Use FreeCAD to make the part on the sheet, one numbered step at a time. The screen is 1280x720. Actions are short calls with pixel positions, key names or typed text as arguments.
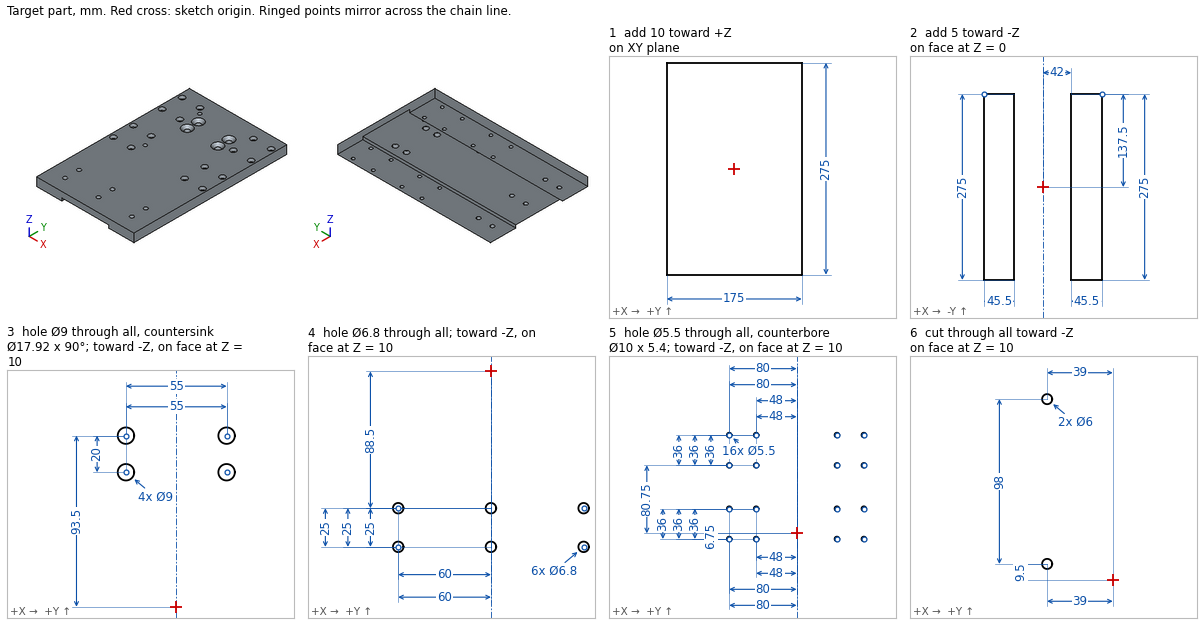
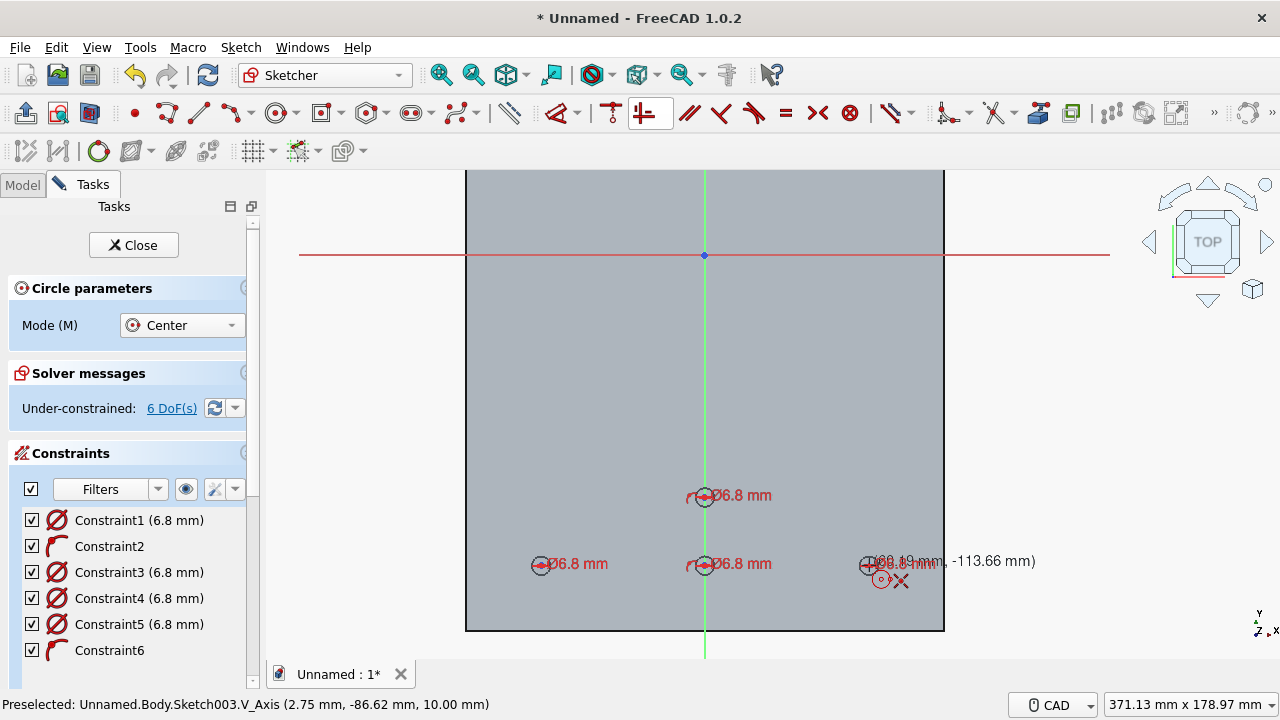
scroll(541, 497, up, 5)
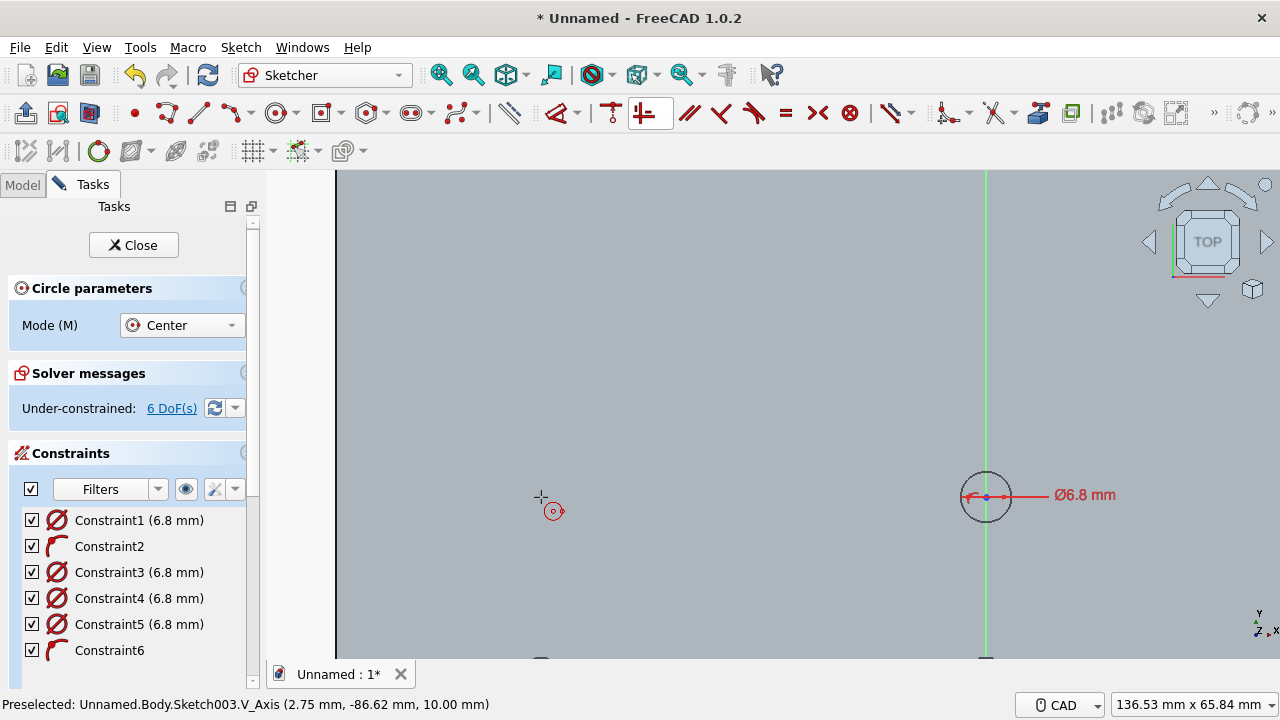
click(541, 496)
move(558, 478)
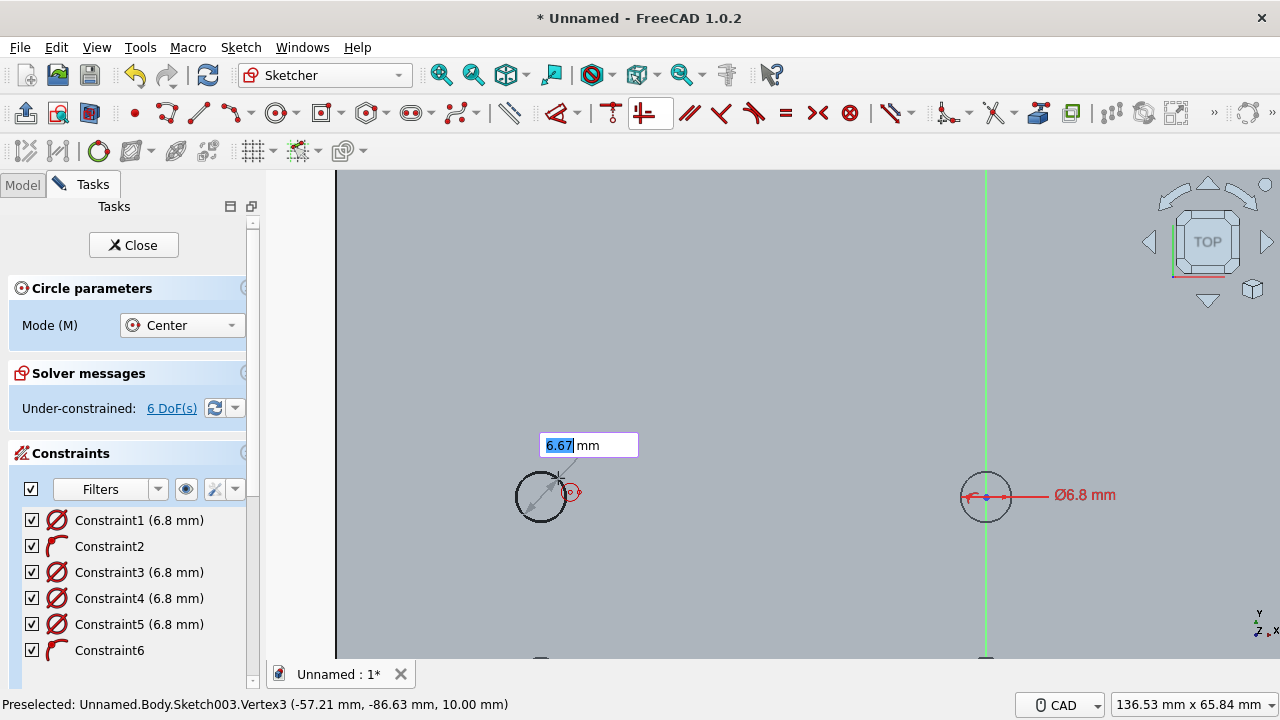
text(6.8)
key(Return)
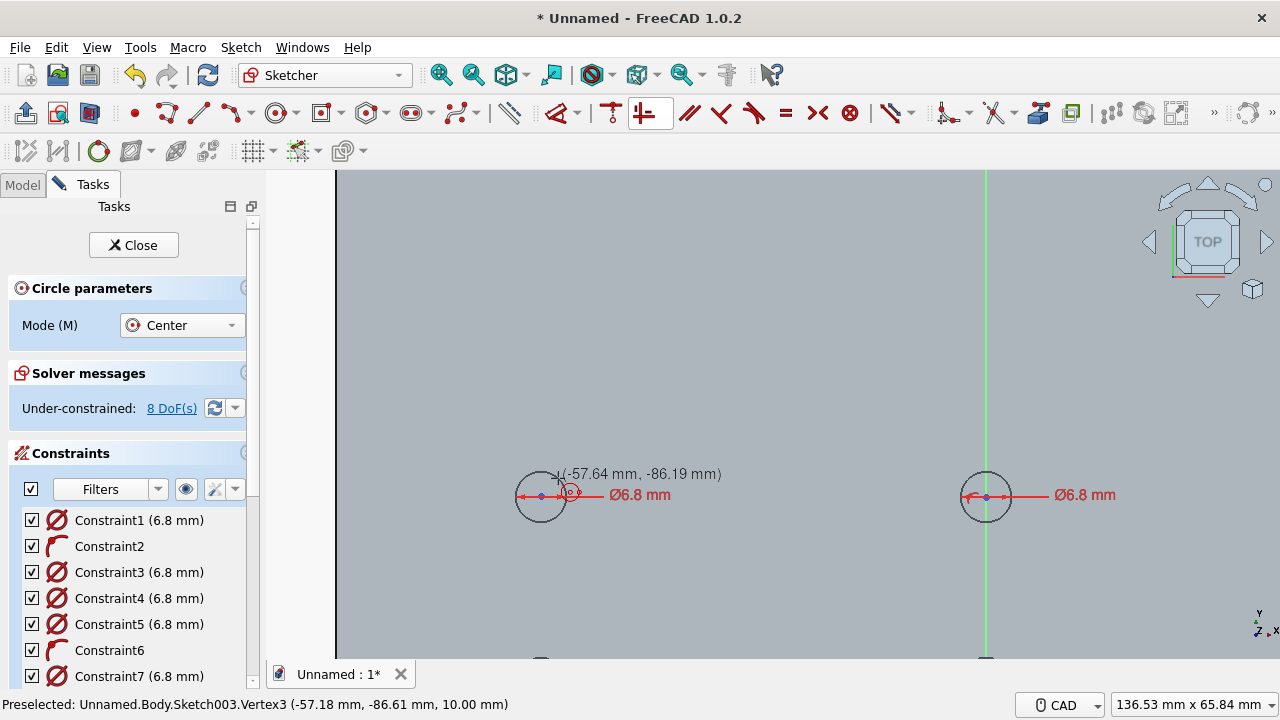
scroll(541, 497, down, 5)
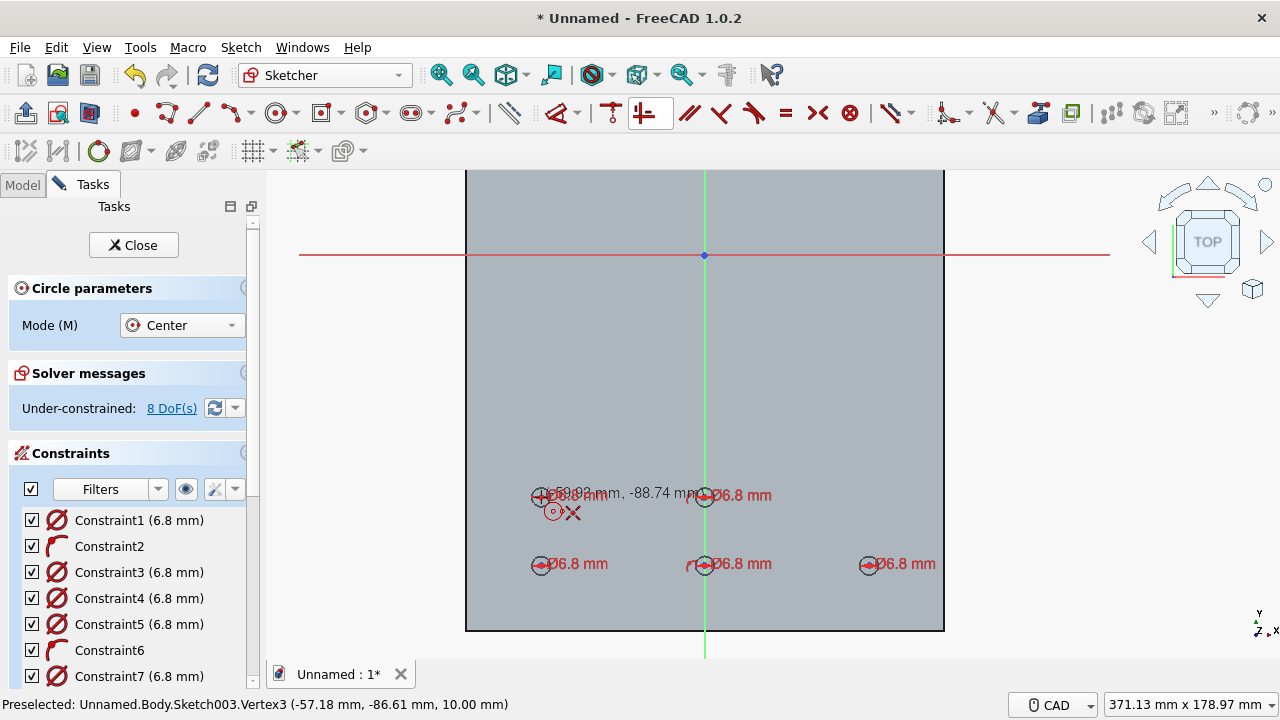
scroll(869, 497, up, 5)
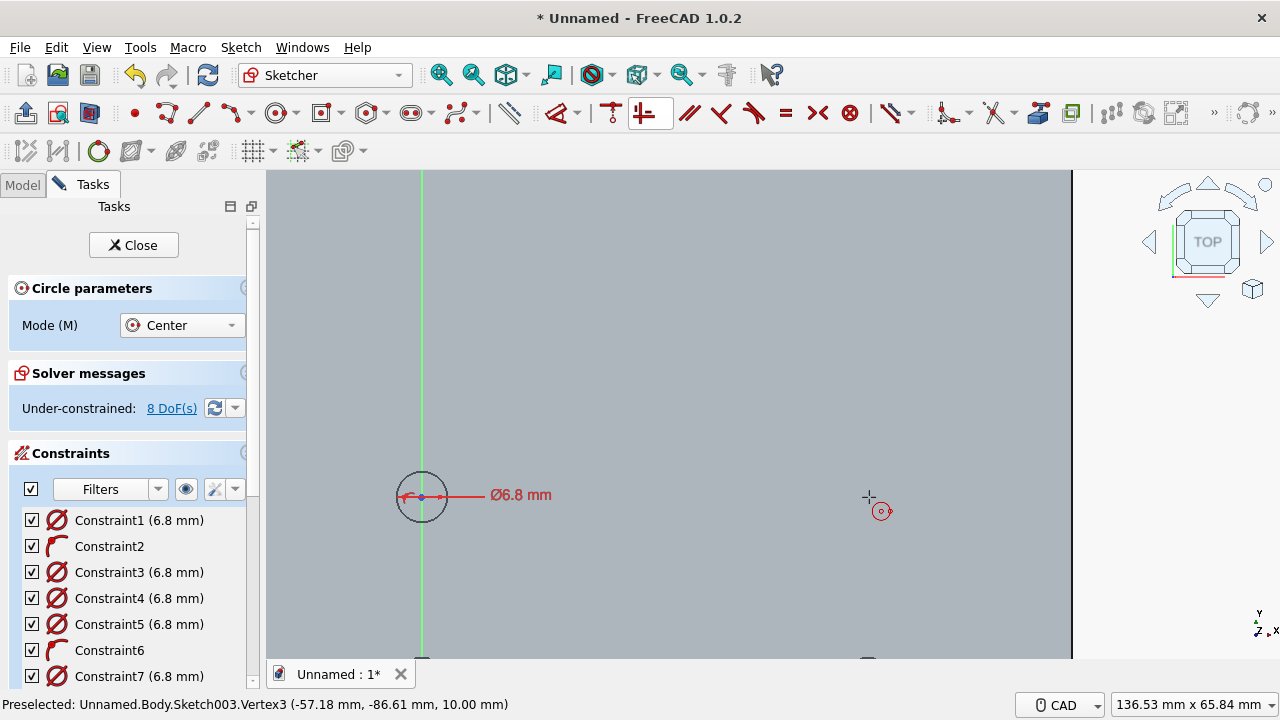
click(868, 496)
move(885, 478)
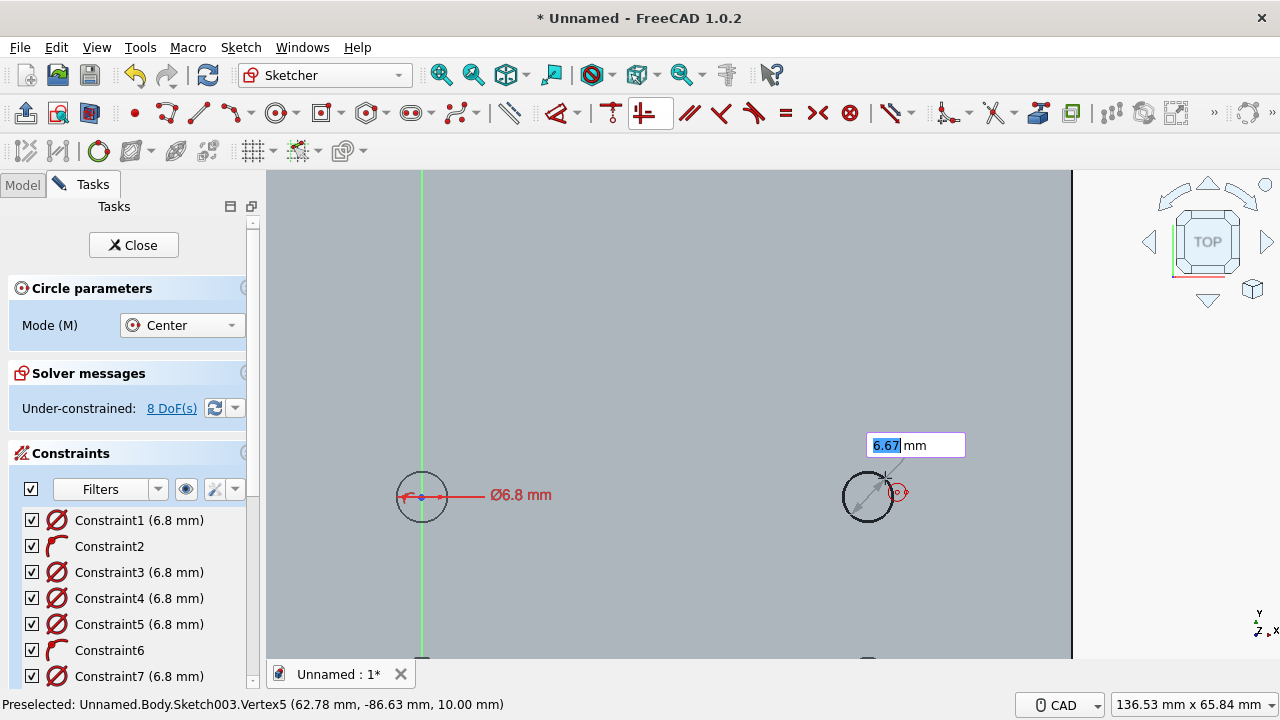
text(6.8)
key(Return)
key(Escape)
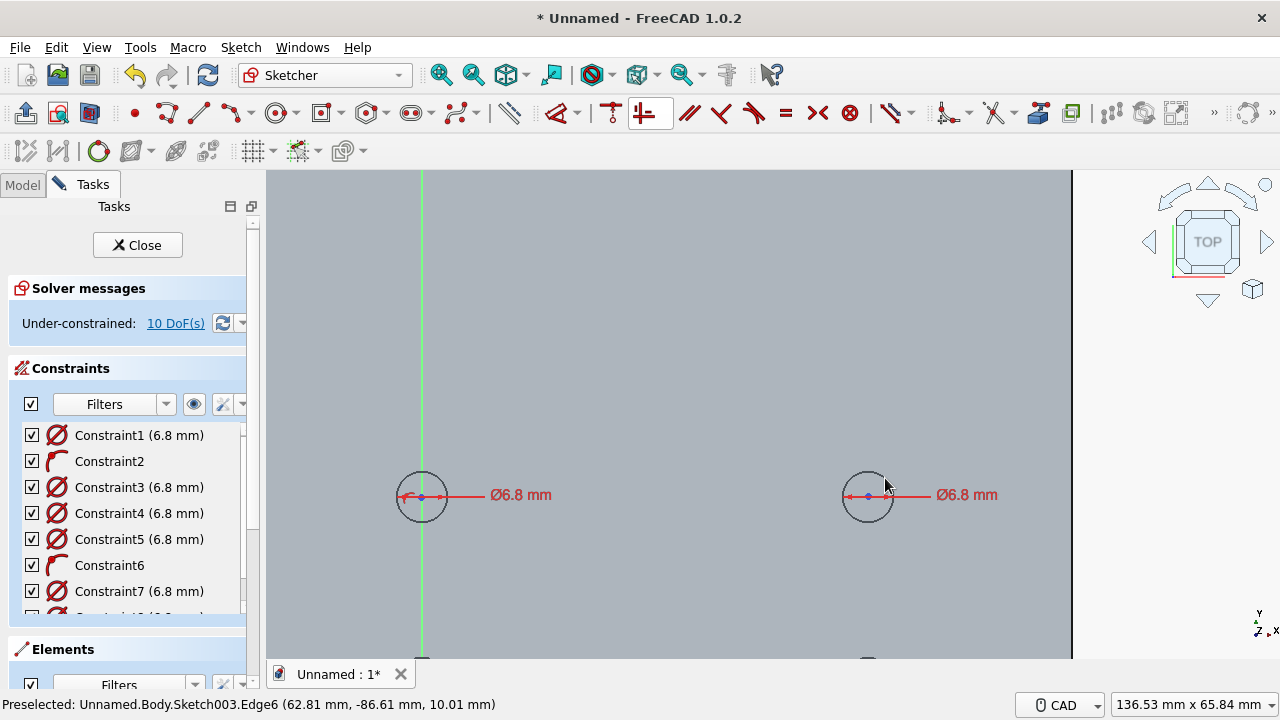
scroll(869, 497, down, 5)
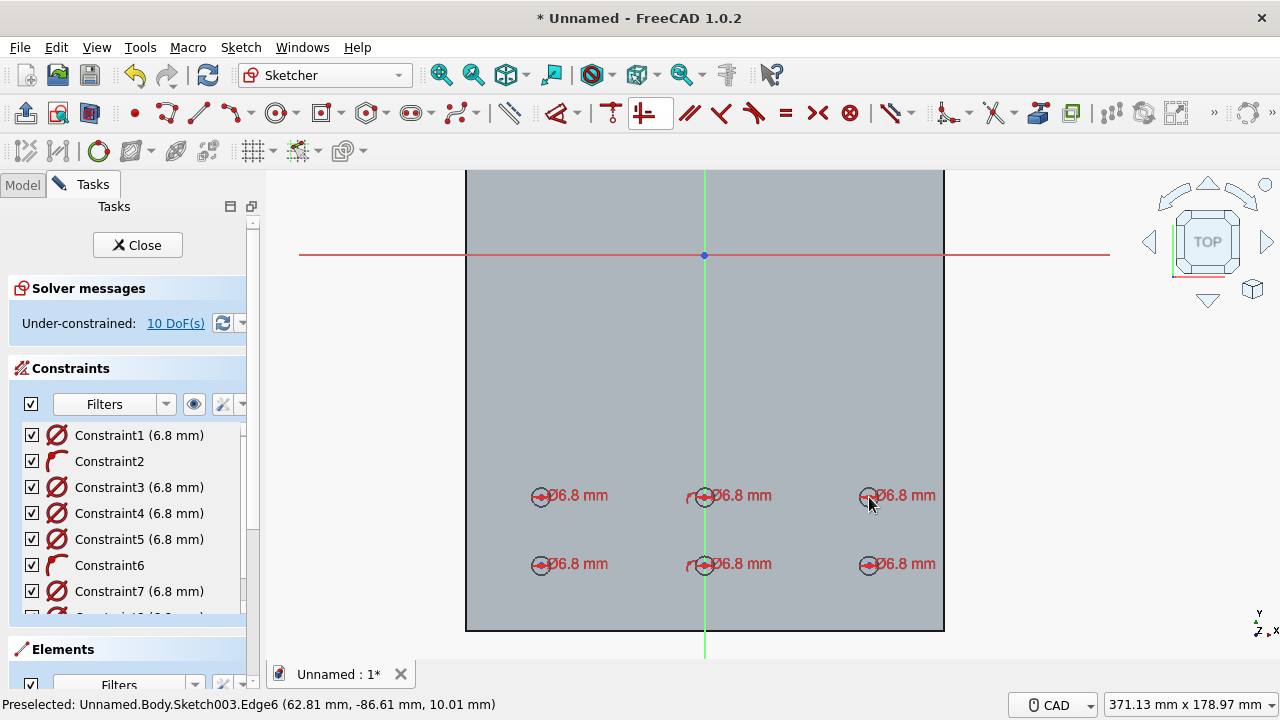
click(541, 566)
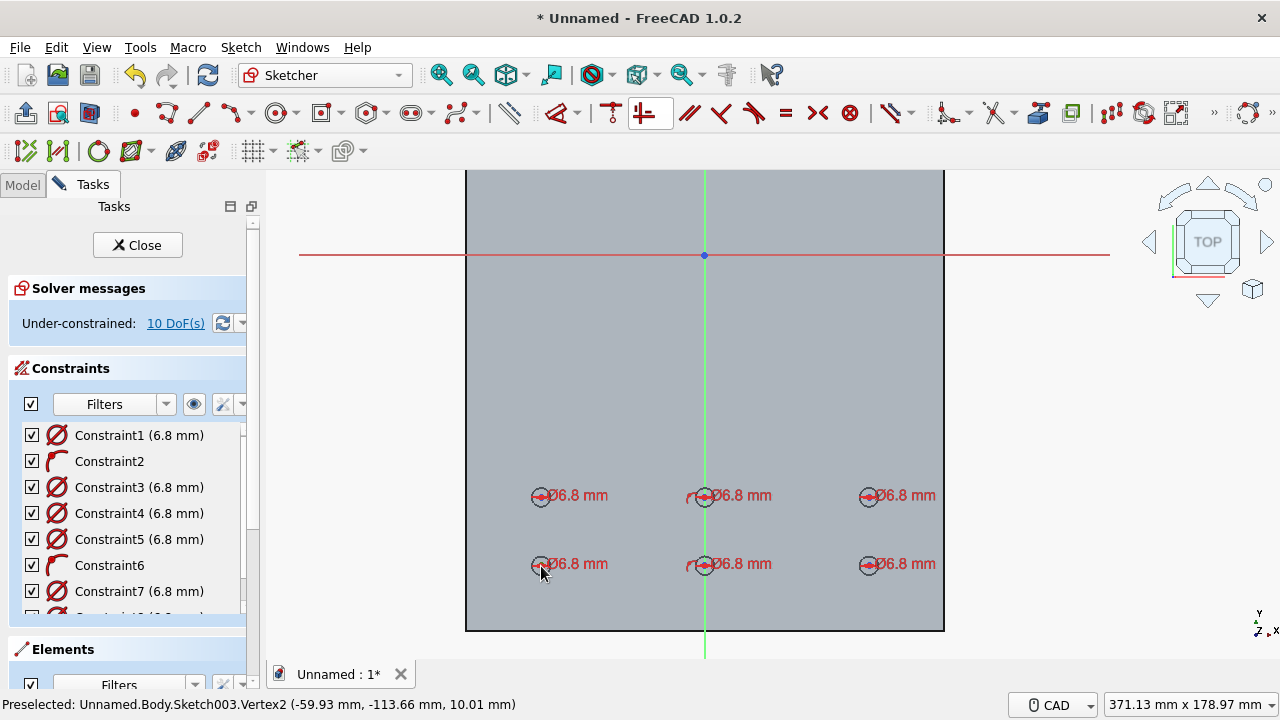
click(869, 566)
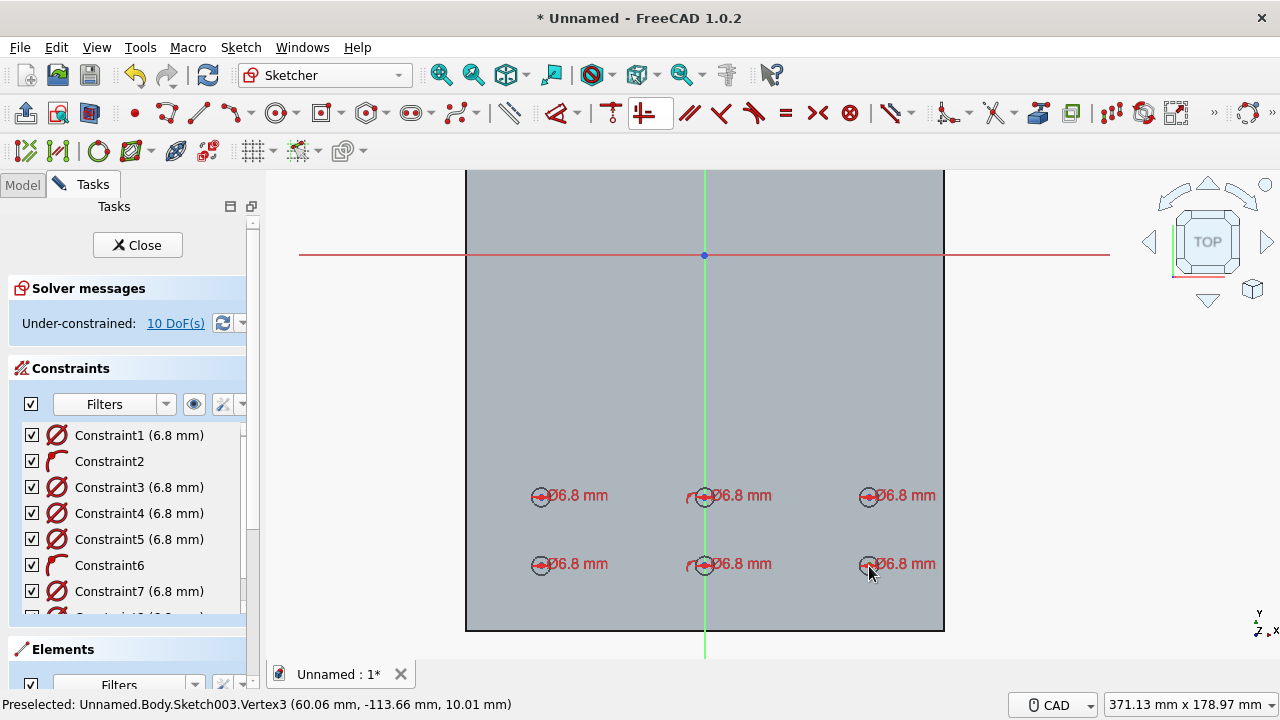
click(705, 445)